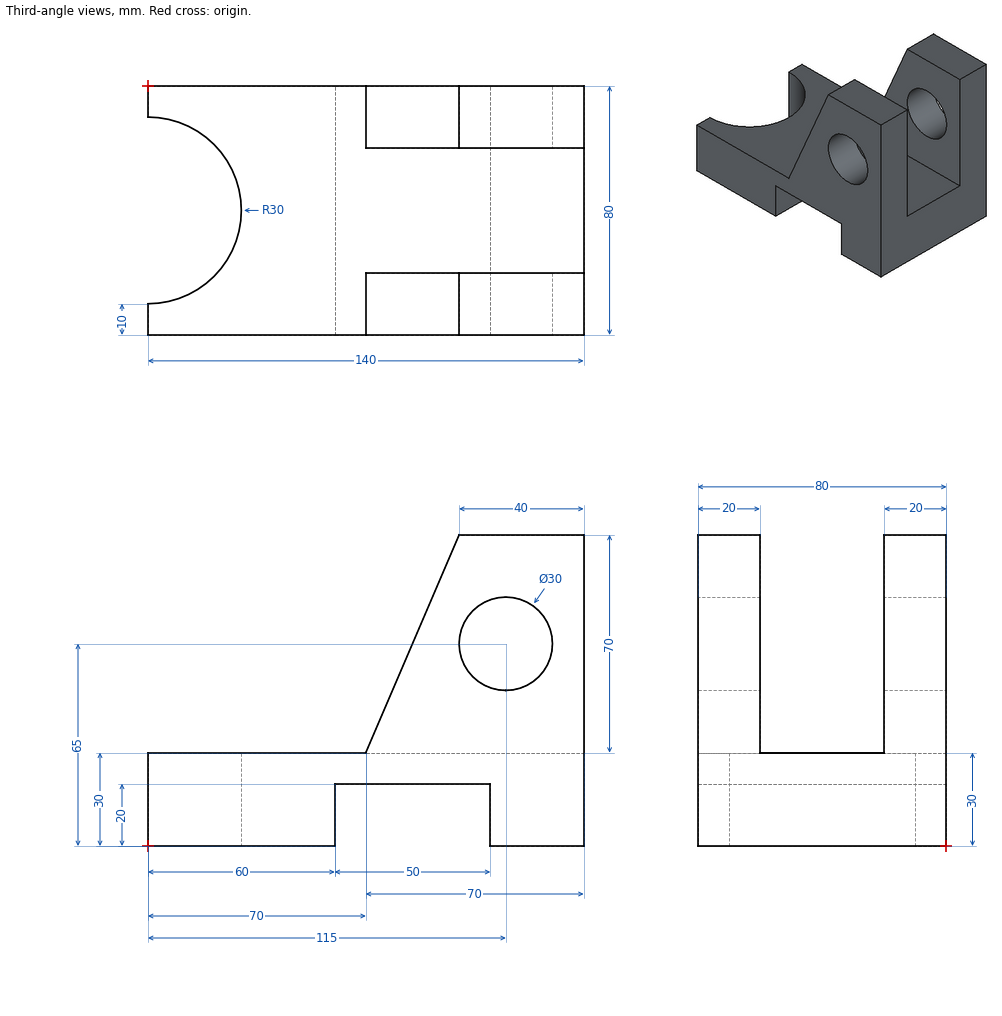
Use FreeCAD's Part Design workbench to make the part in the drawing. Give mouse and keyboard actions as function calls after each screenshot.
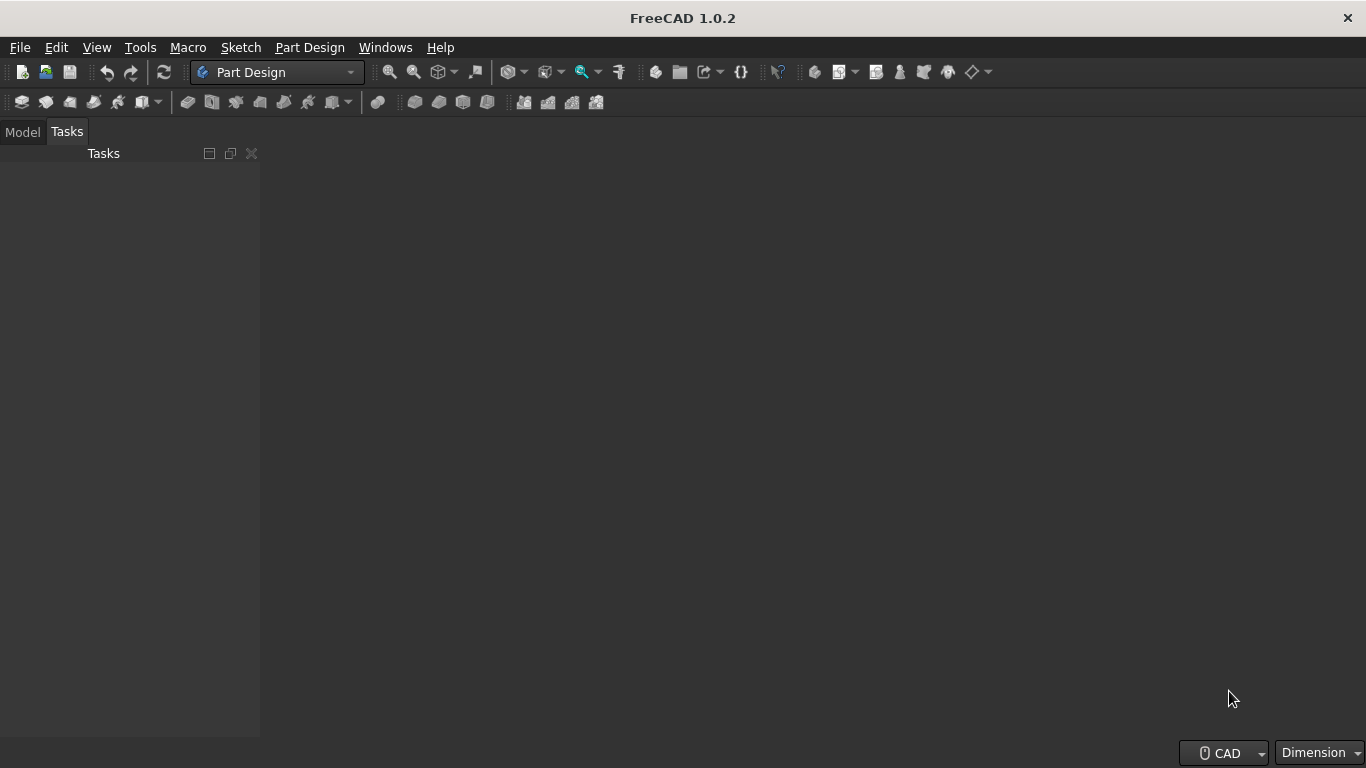
click(22, 72)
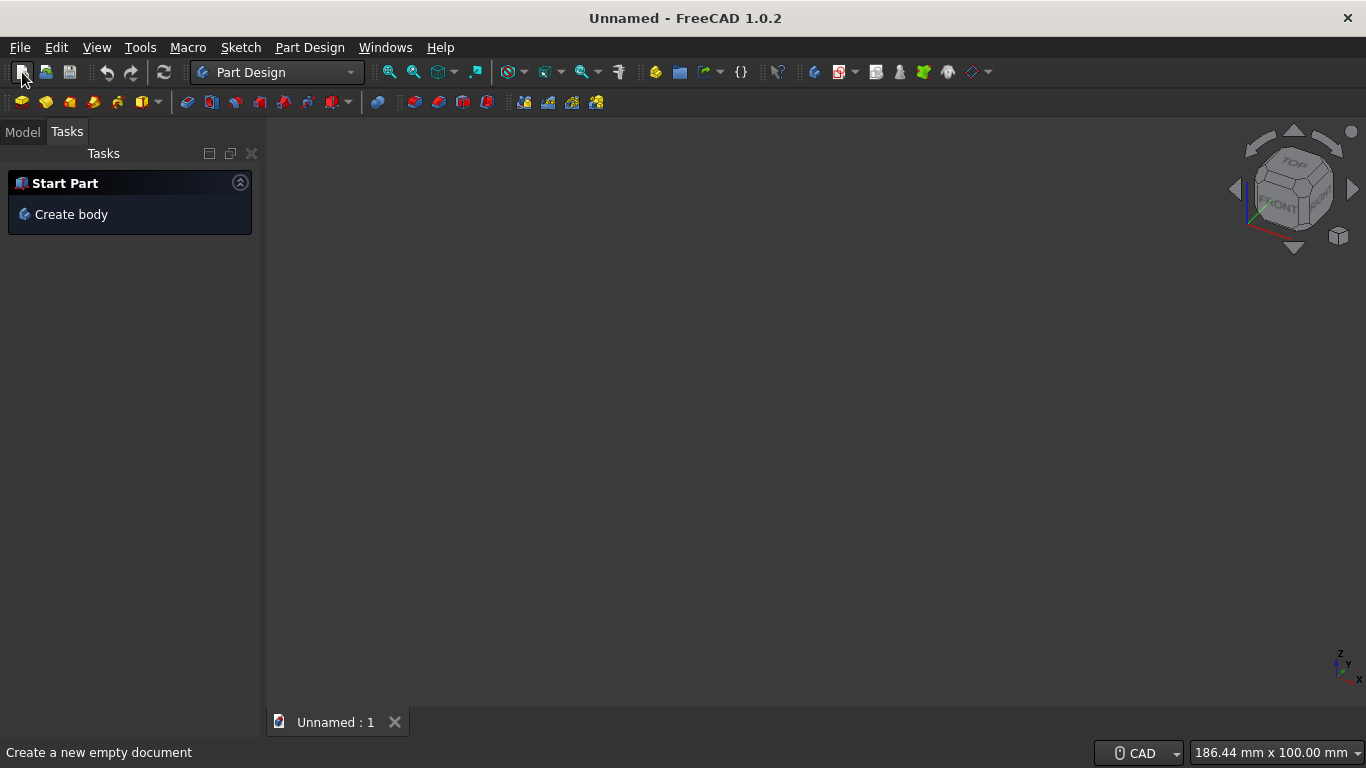
click(840, 72)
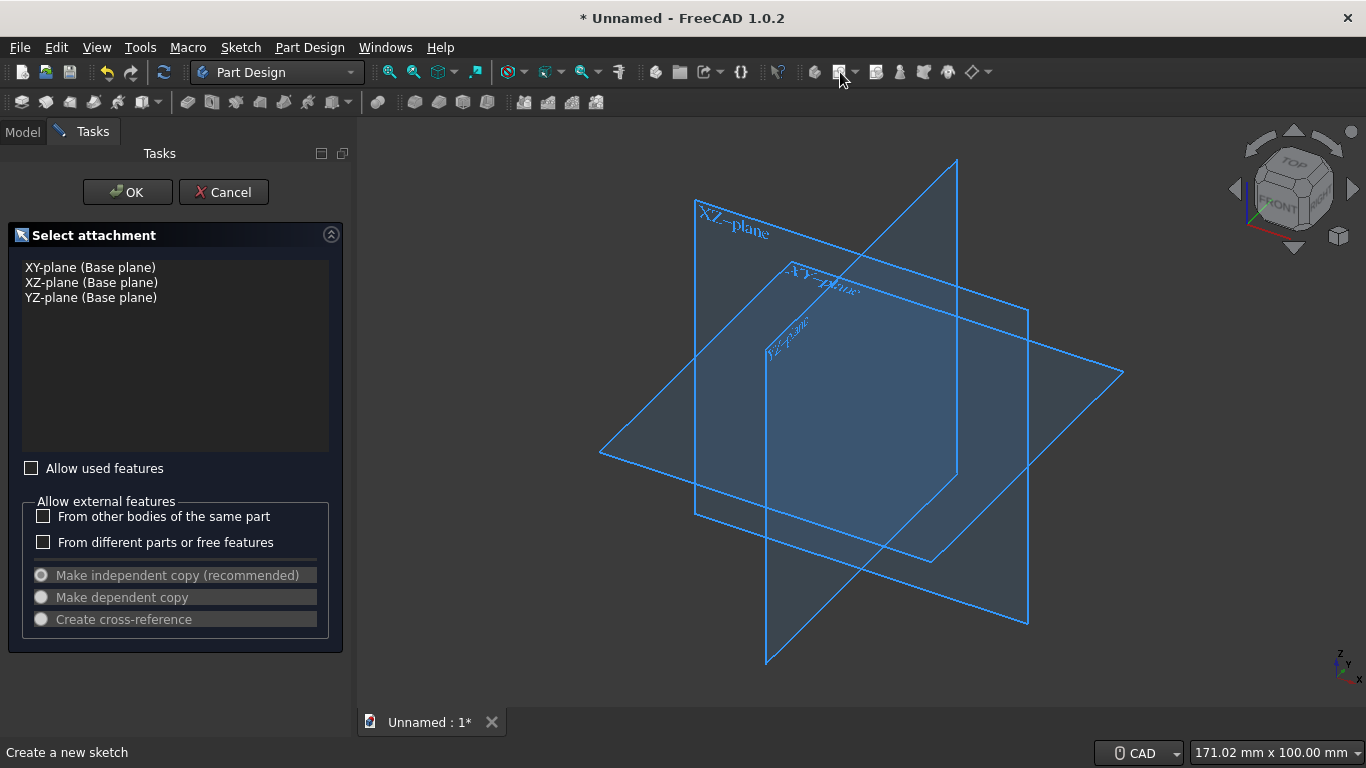
click(82, 268)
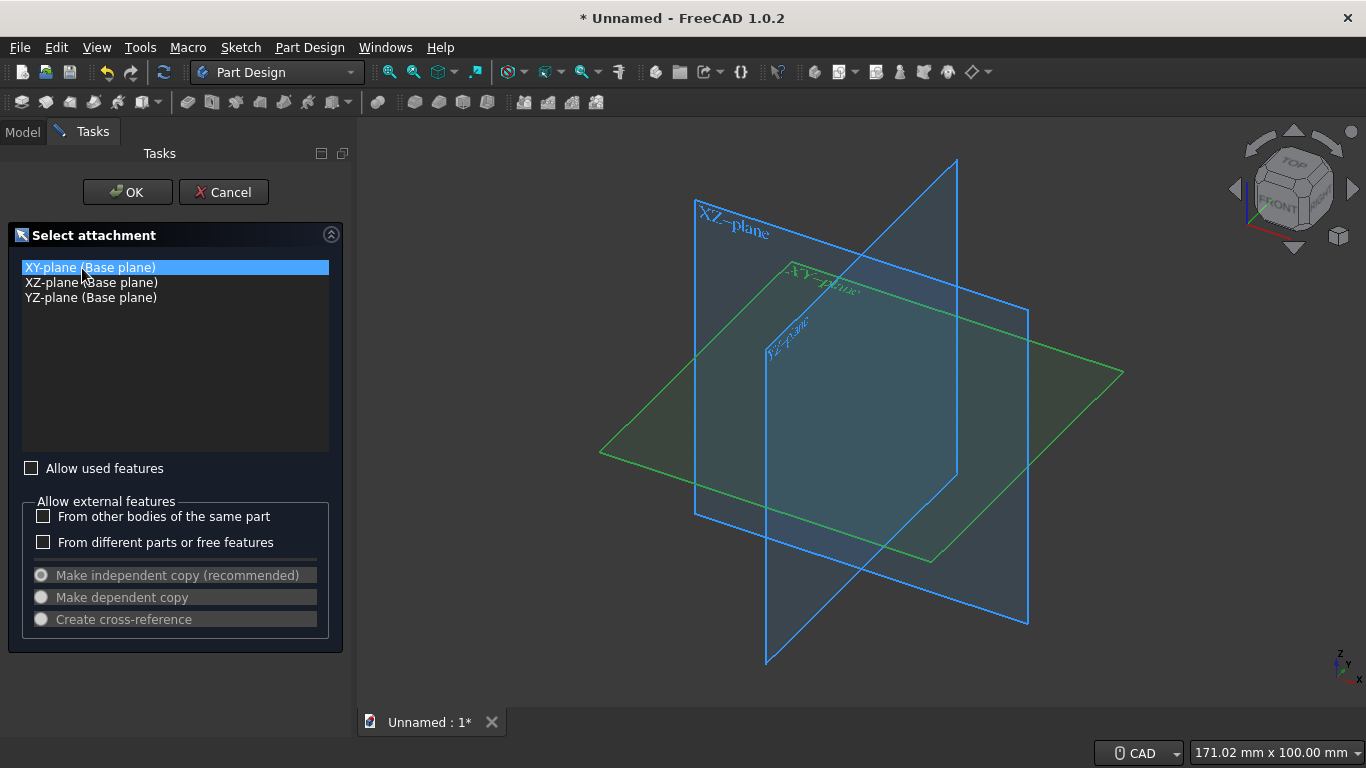
click(128, 192)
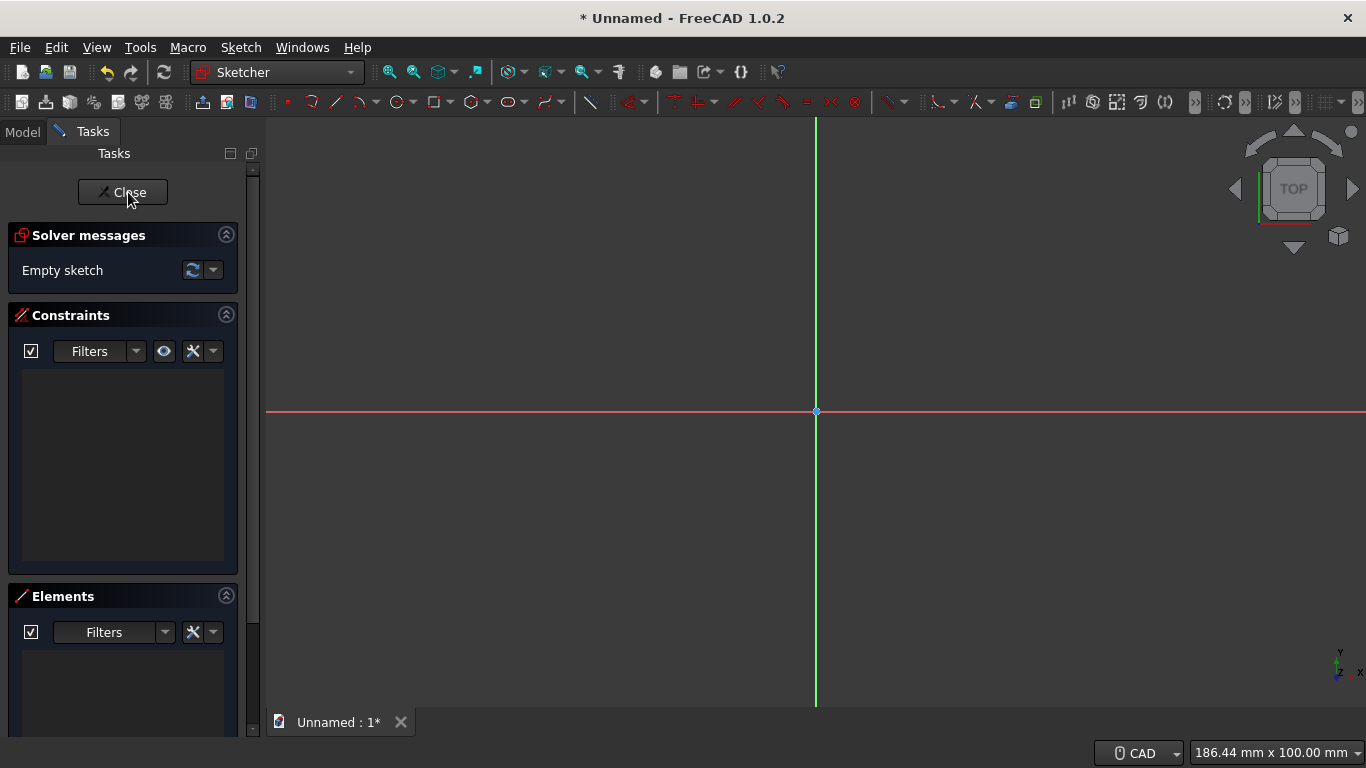
scroll(294, 145, down, 3)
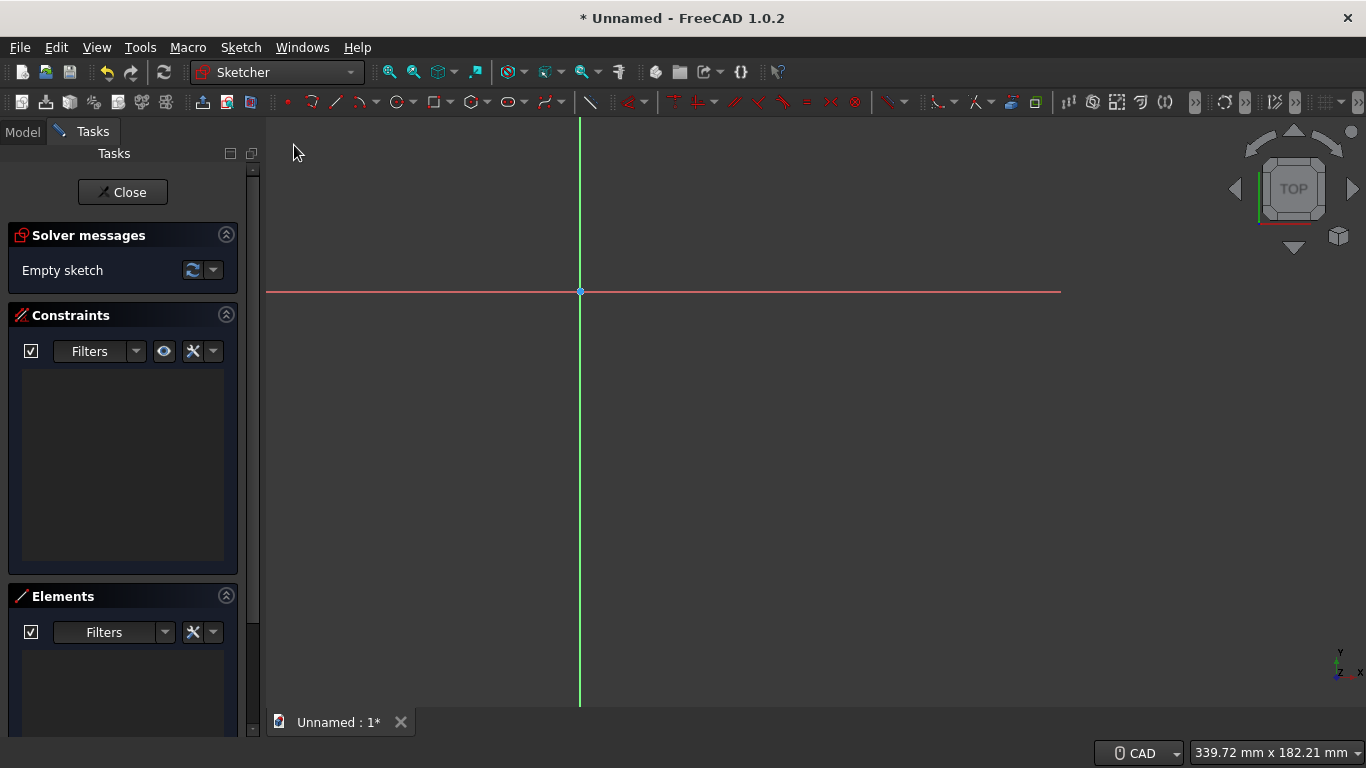
scroll(928, 440, up, 2)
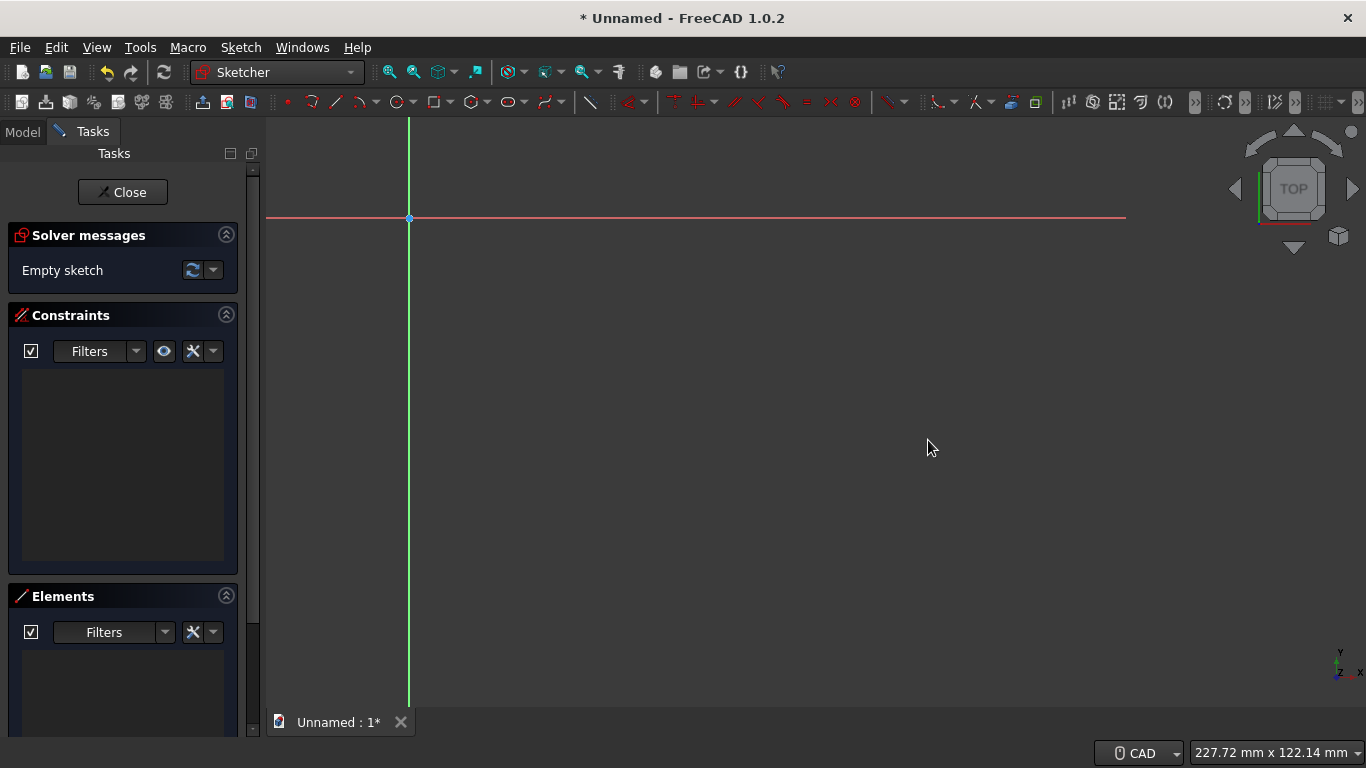
click(312, 102)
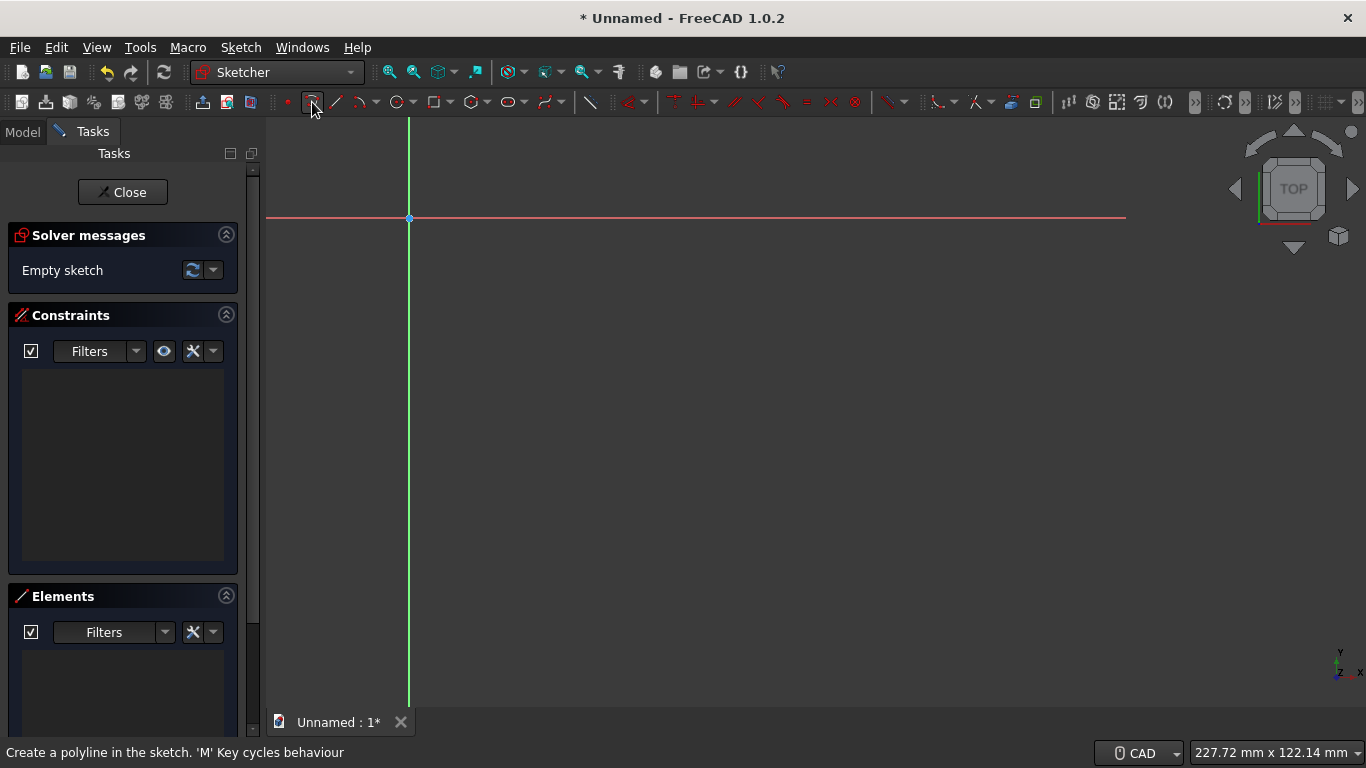
click(409, 556)
click(418, 605)
click(1086, 605)
click(1086, 218)
click(409, 218)
click(418, 267)
right_click(418, 267)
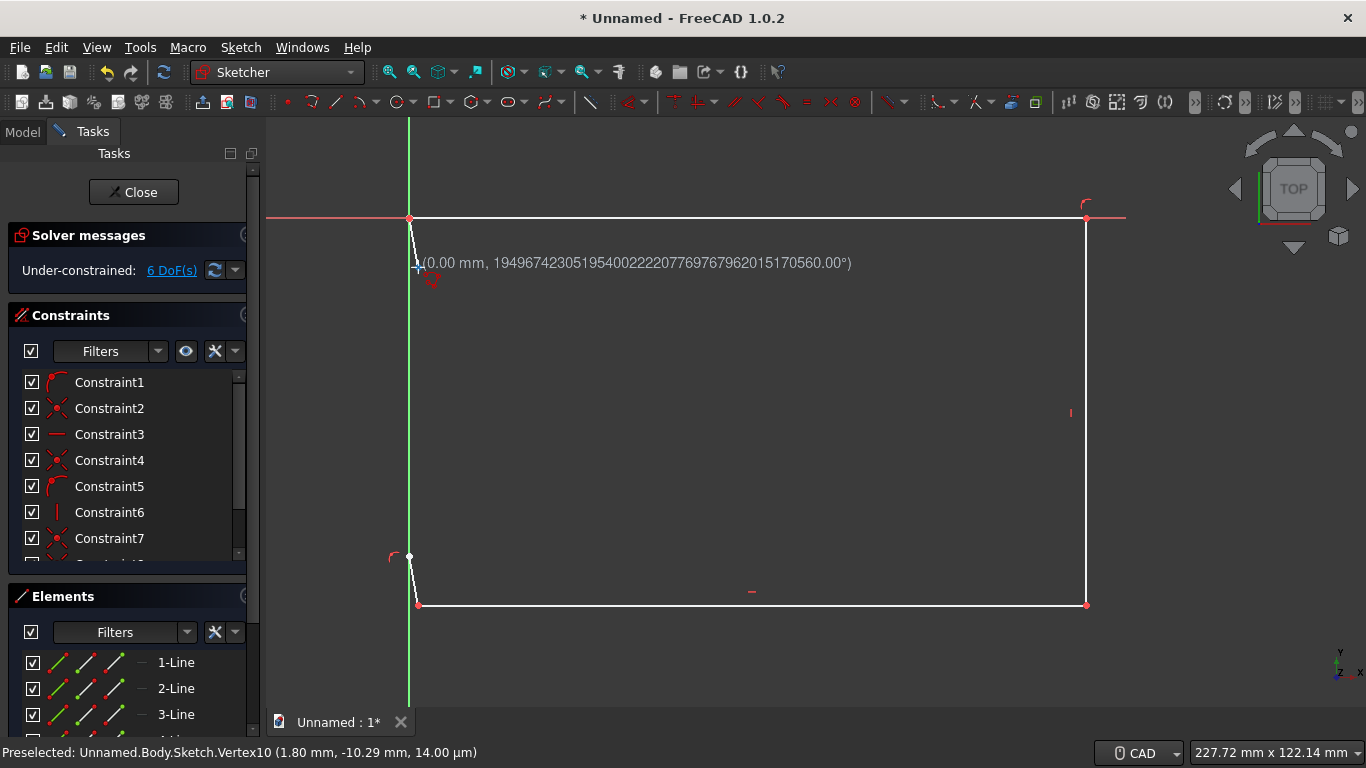
key(g)
key(3)
key(a)